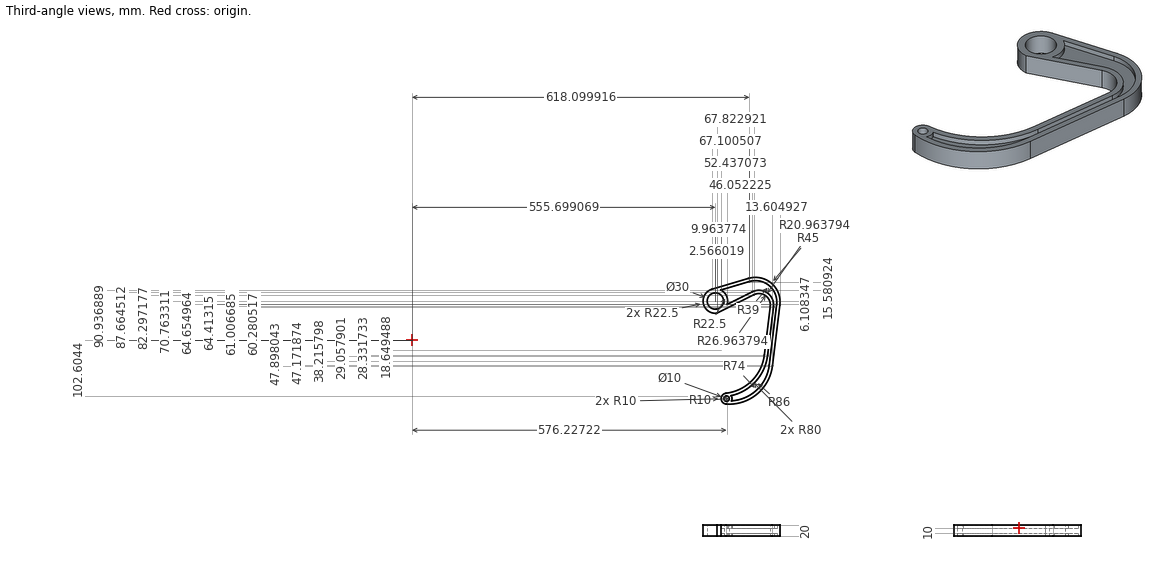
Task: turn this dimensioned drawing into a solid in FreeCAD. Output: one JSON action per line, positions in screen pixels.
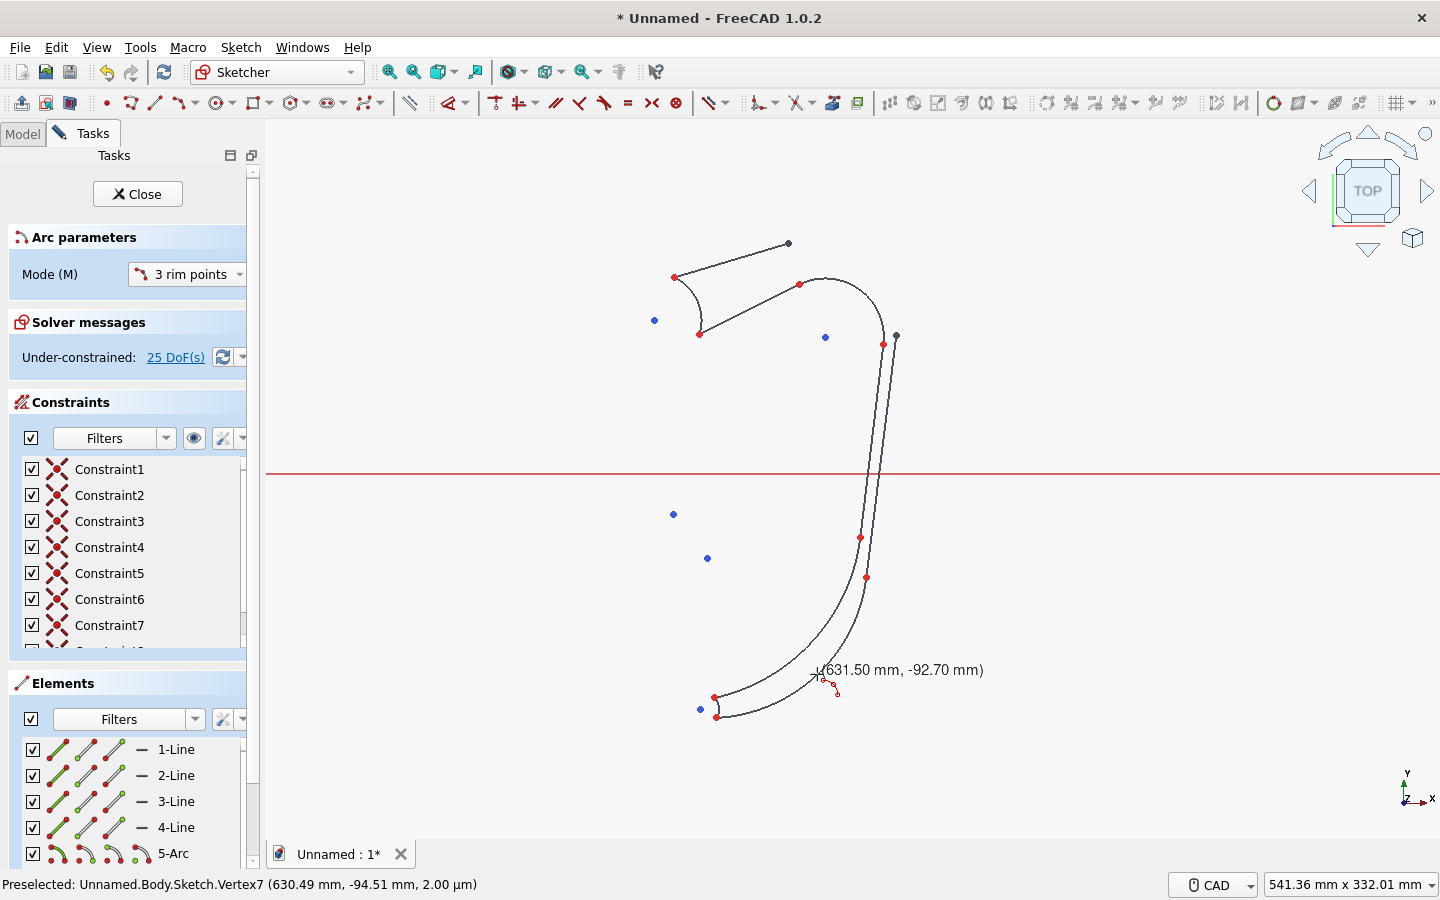
{"action": "scroll", "coordinate": [896, 334], "scroll_direction": "up", "scroll_amount": 2}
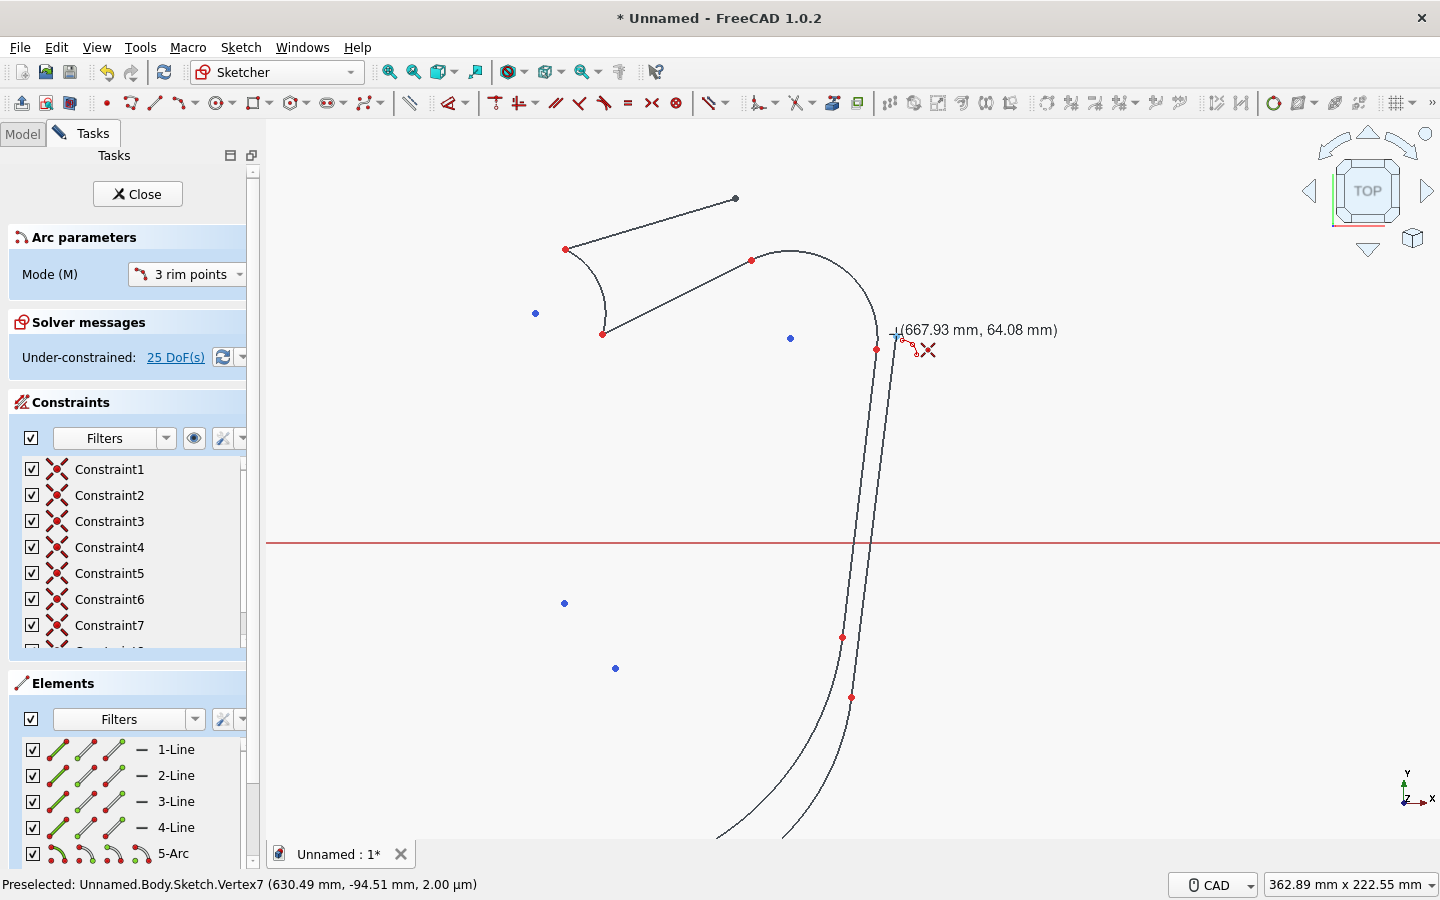
{"action": "left_click", "coordinate": [896, 336]}
{"action": "left_click", "coordinate": [735, 199]}
{"action": "left_click", "coordinate": [852, 223]}
{"action": "key", "text": "Escape"}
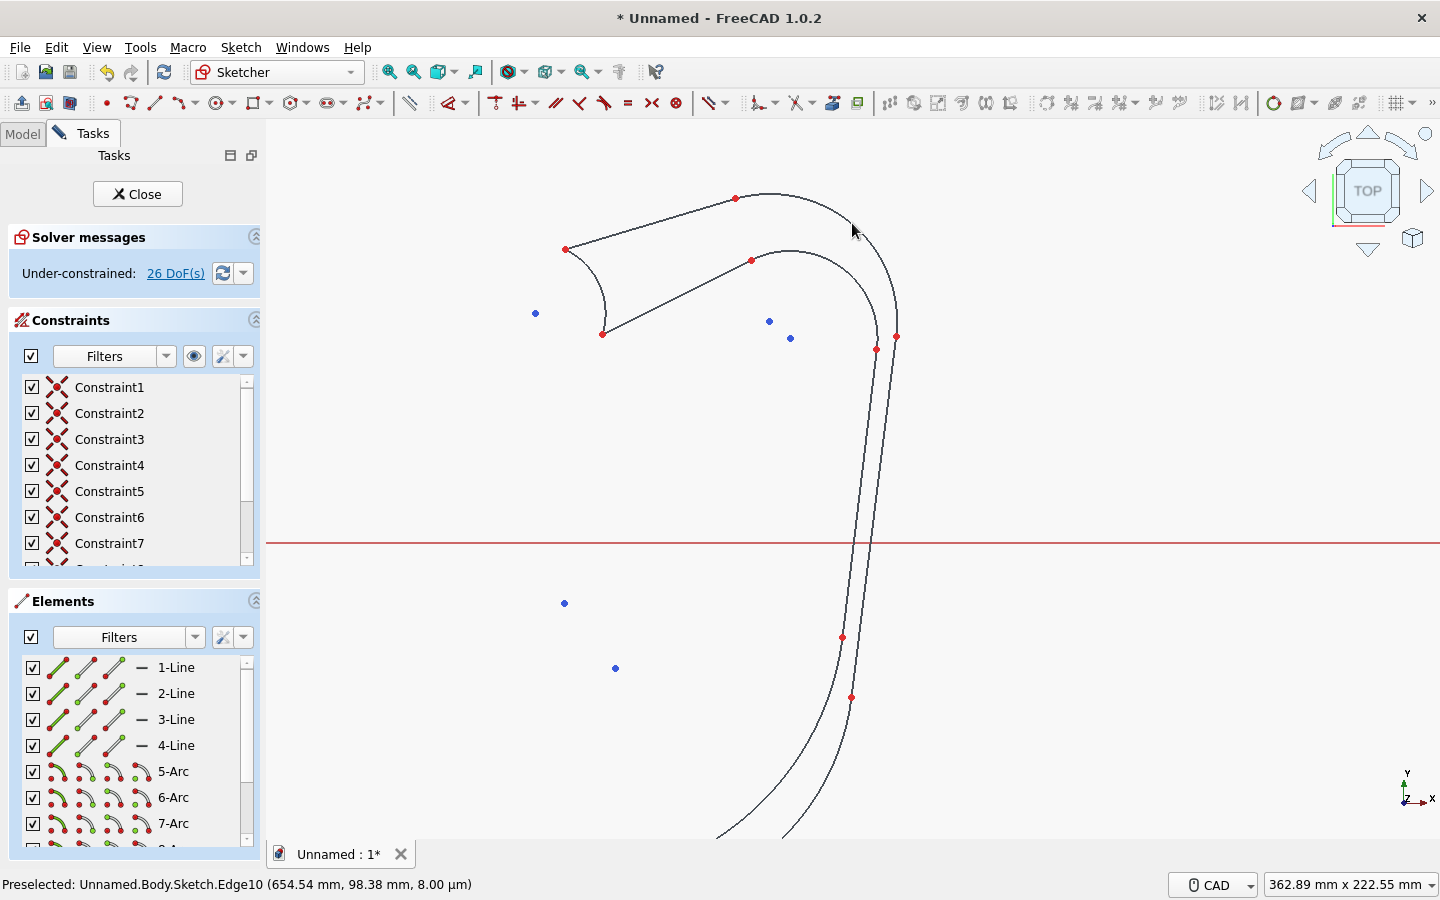
{"action": "left_click", "coordinate": [684, 214]}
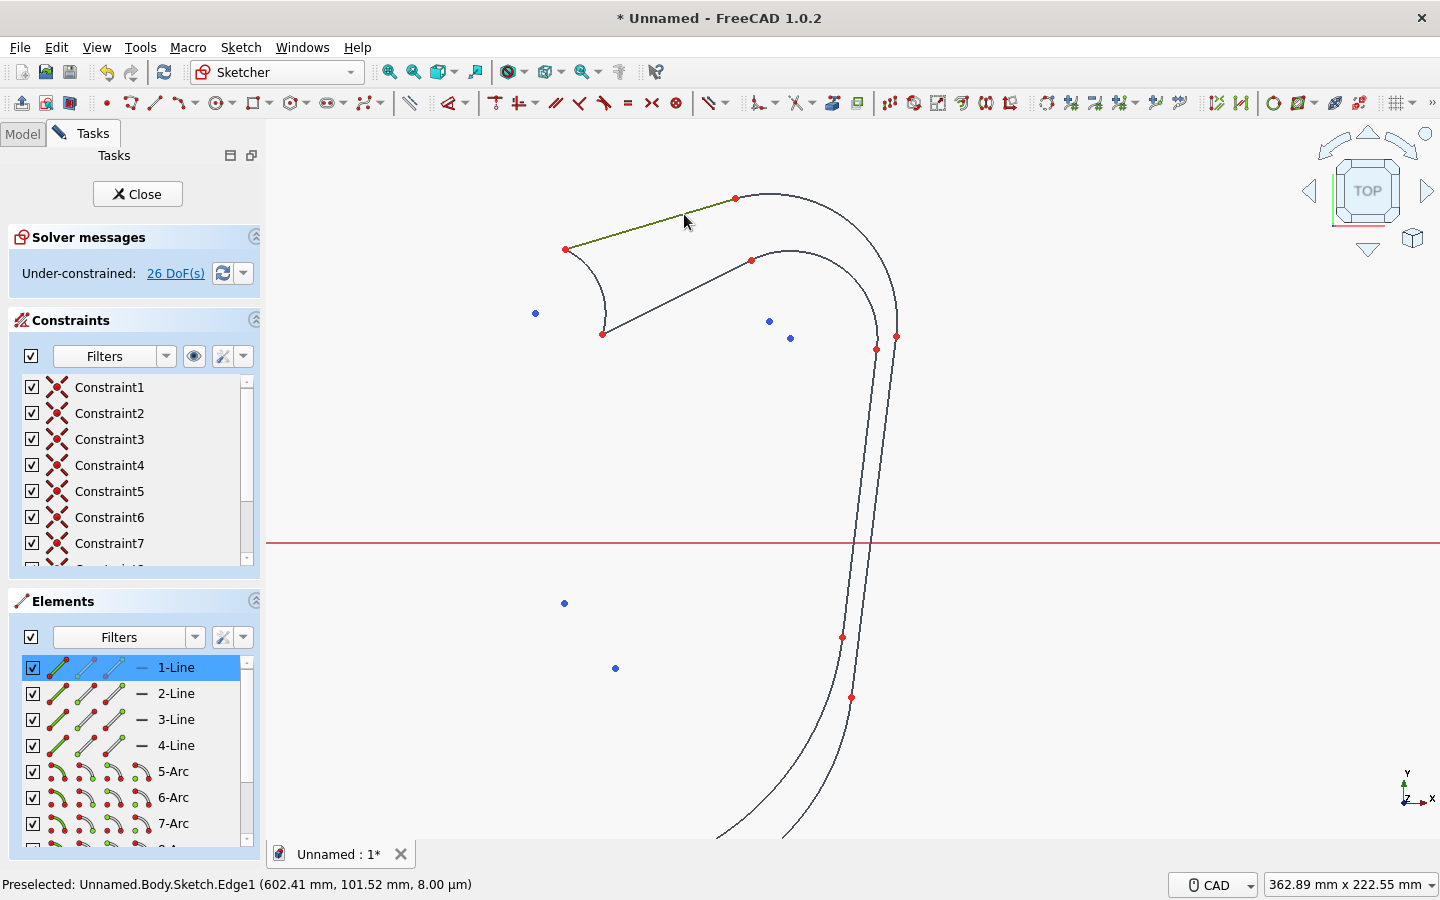
{"action": "left_click", "coordinate": [883, 263]}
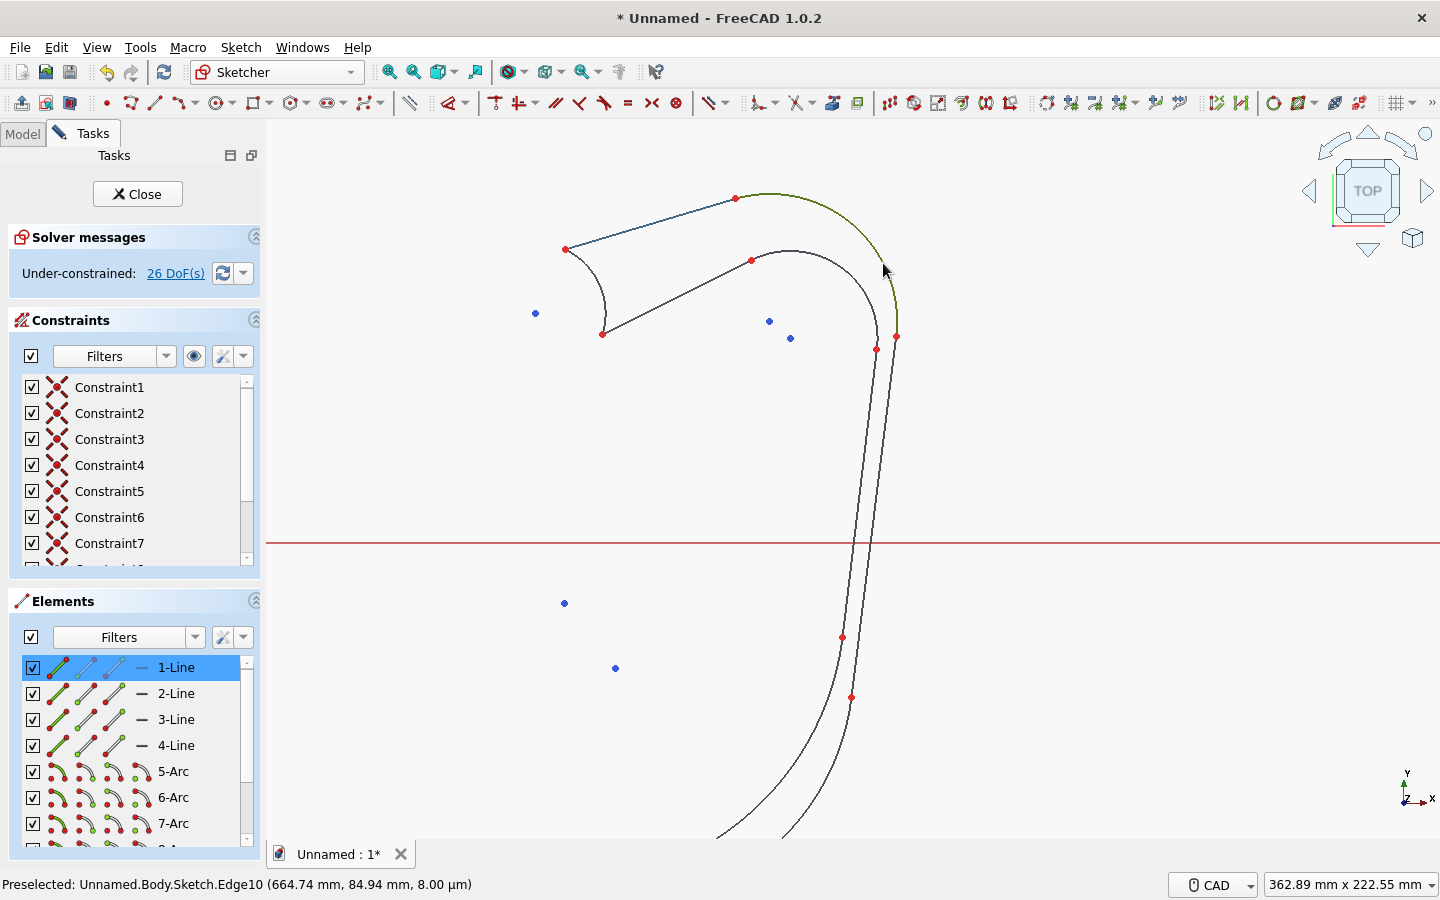
{"action": "left_click", "coordinate": [604, 104]}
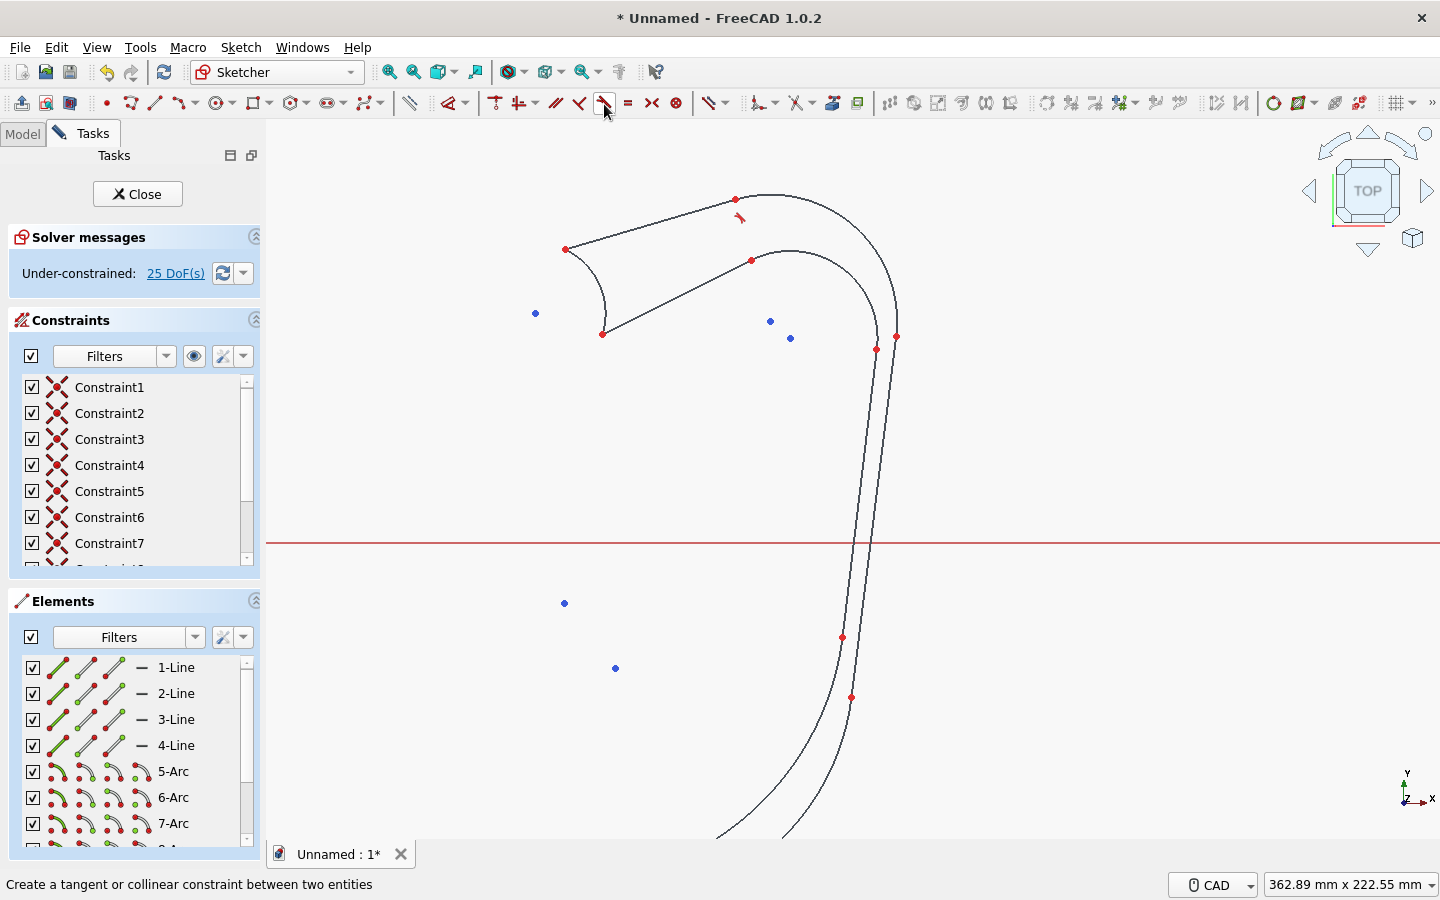
{"action": "left_click", "coordinate": [647, 312]}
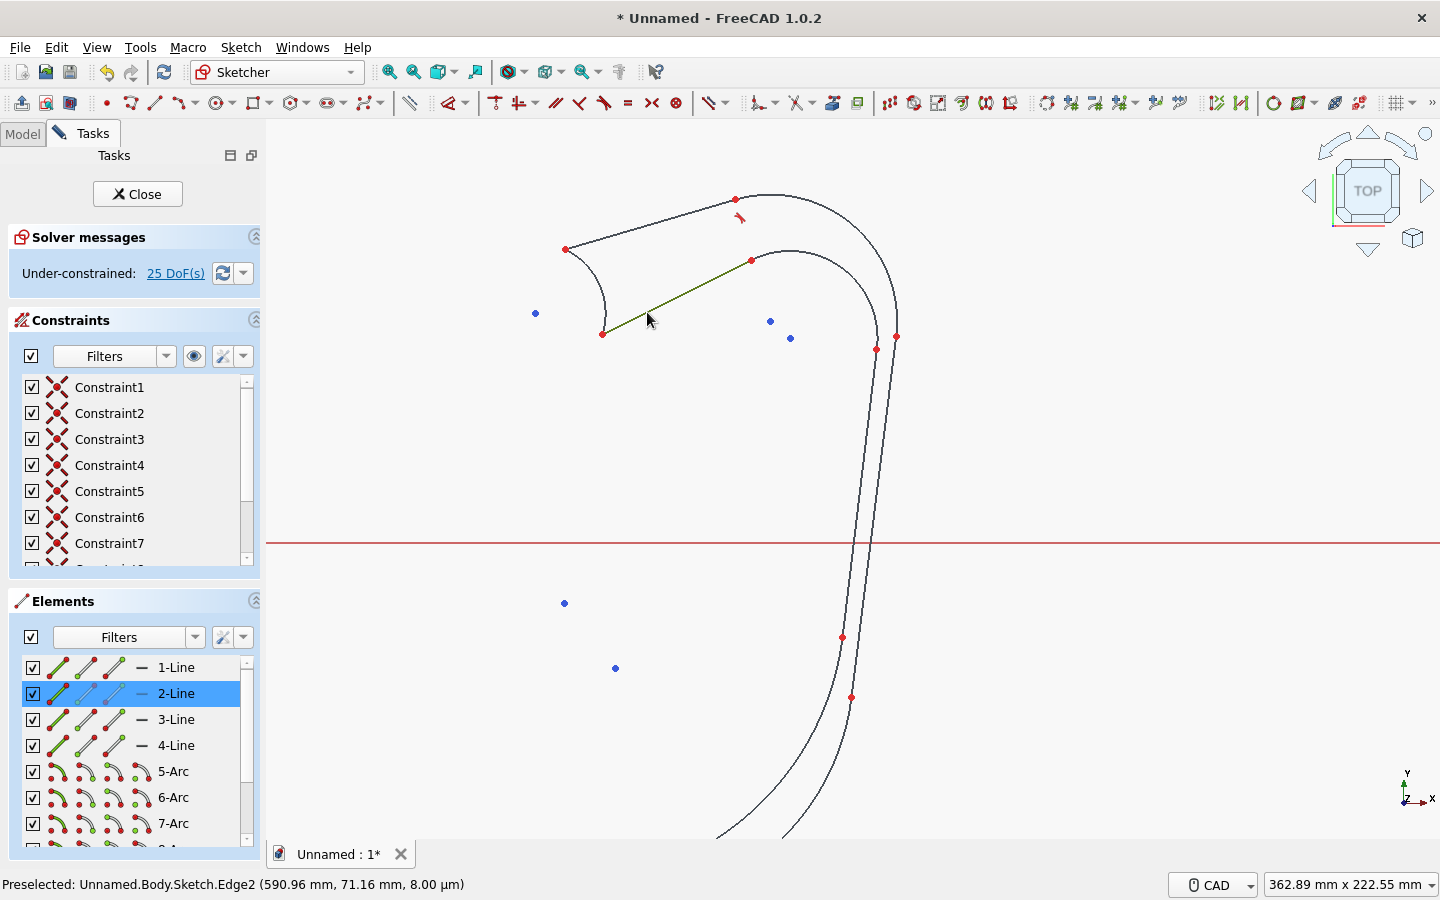
{"action": "left_click", "coordinate": [866, 295]}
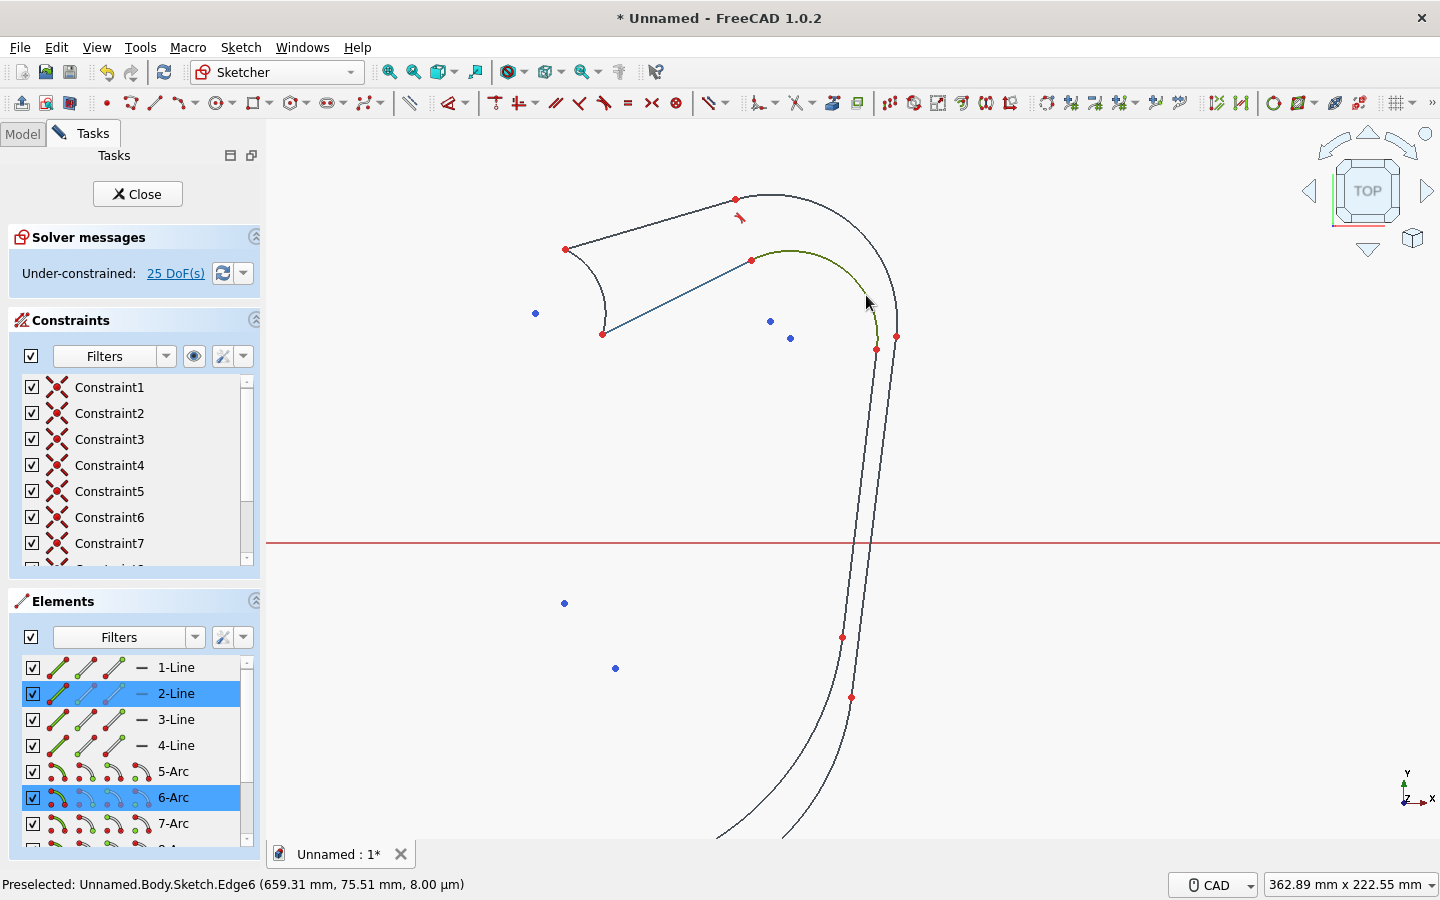
{"action": "key", "text": "t"}